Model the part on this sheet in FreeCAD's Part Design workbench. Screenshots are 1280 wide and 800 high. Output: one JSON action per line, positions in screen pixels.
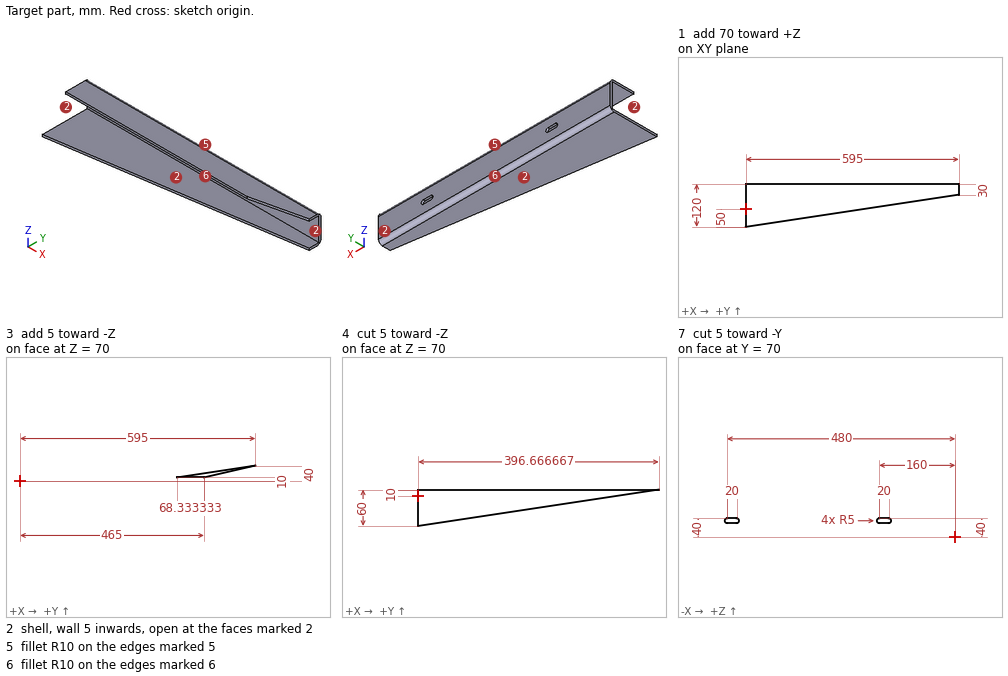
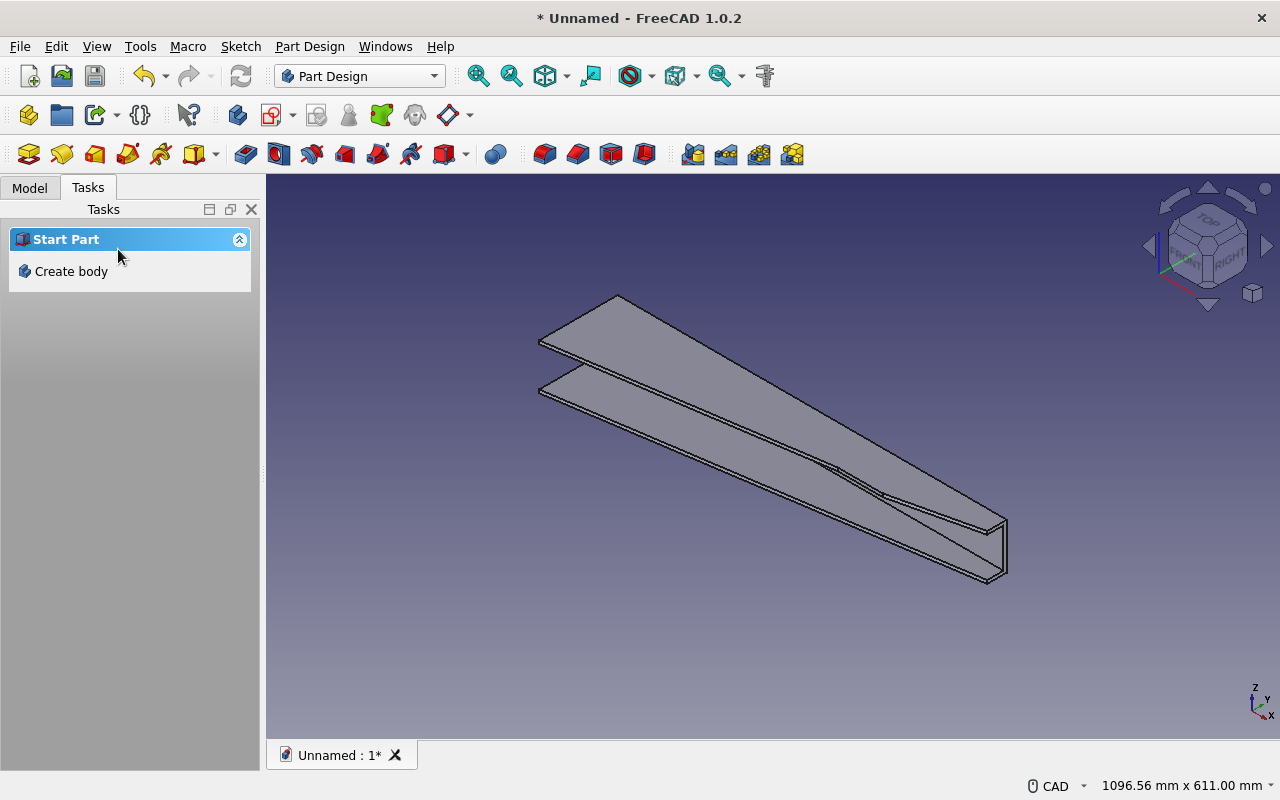
{"action": "left_click", "coordinate": [729, 391]}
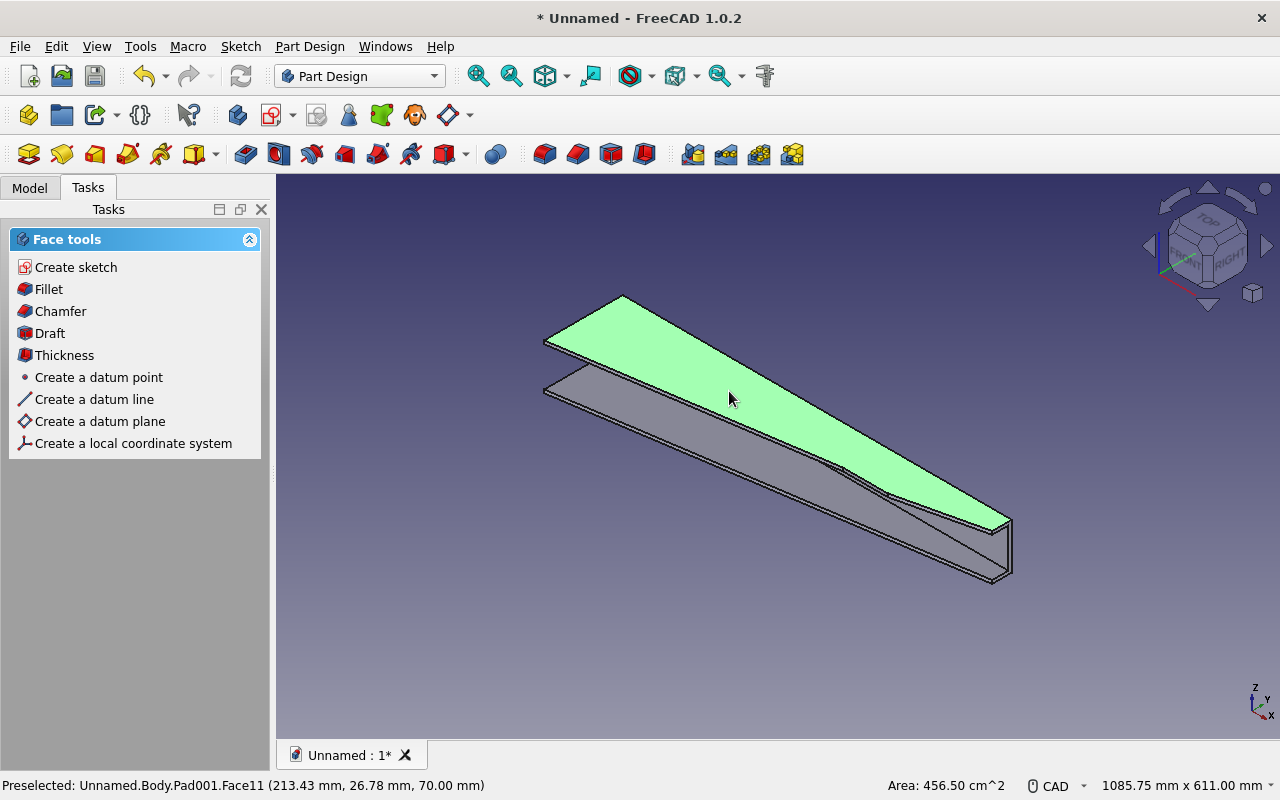
{"action": "left_click", "coordinate": [270, 116]}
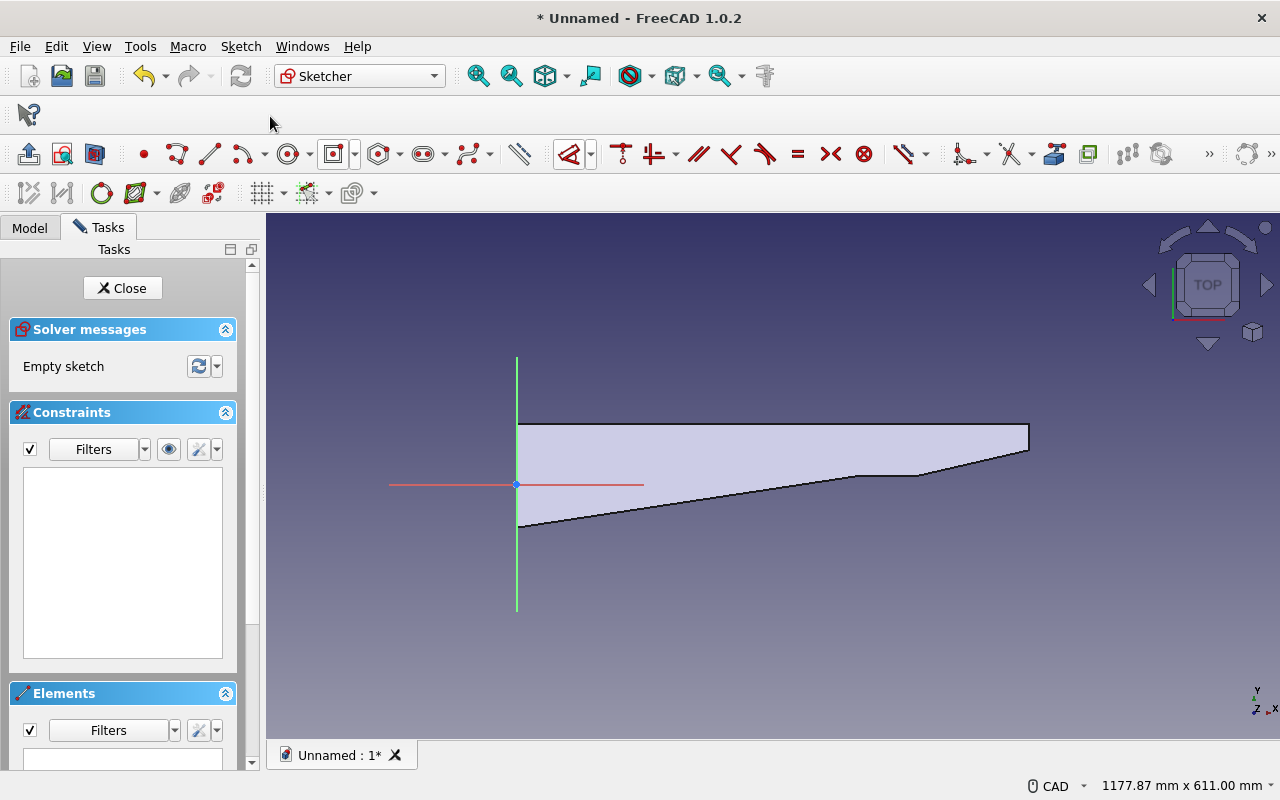
{"action": "scroll", "coordinate": [667, 533], "scroll_direction": "up", "scroll_amount": 3}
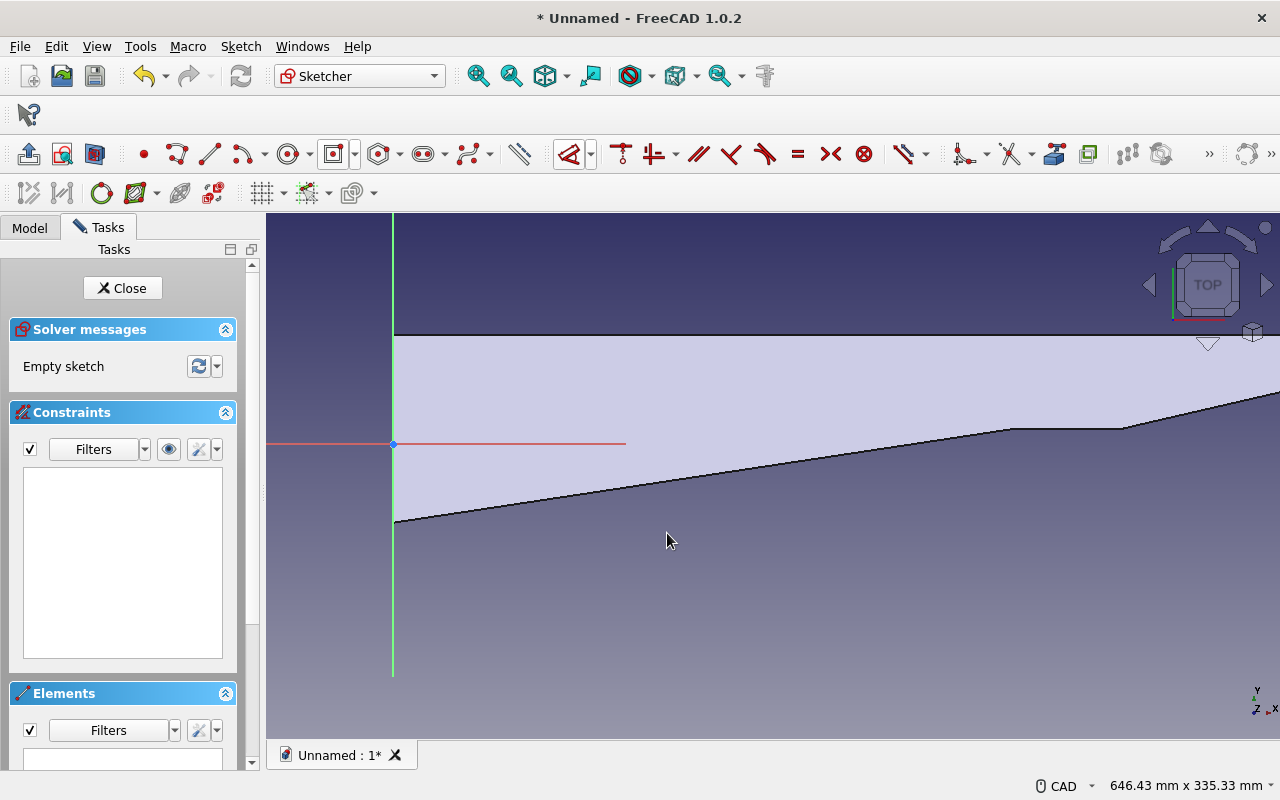
{"action": "left_click", "coordinate": [177, 154]}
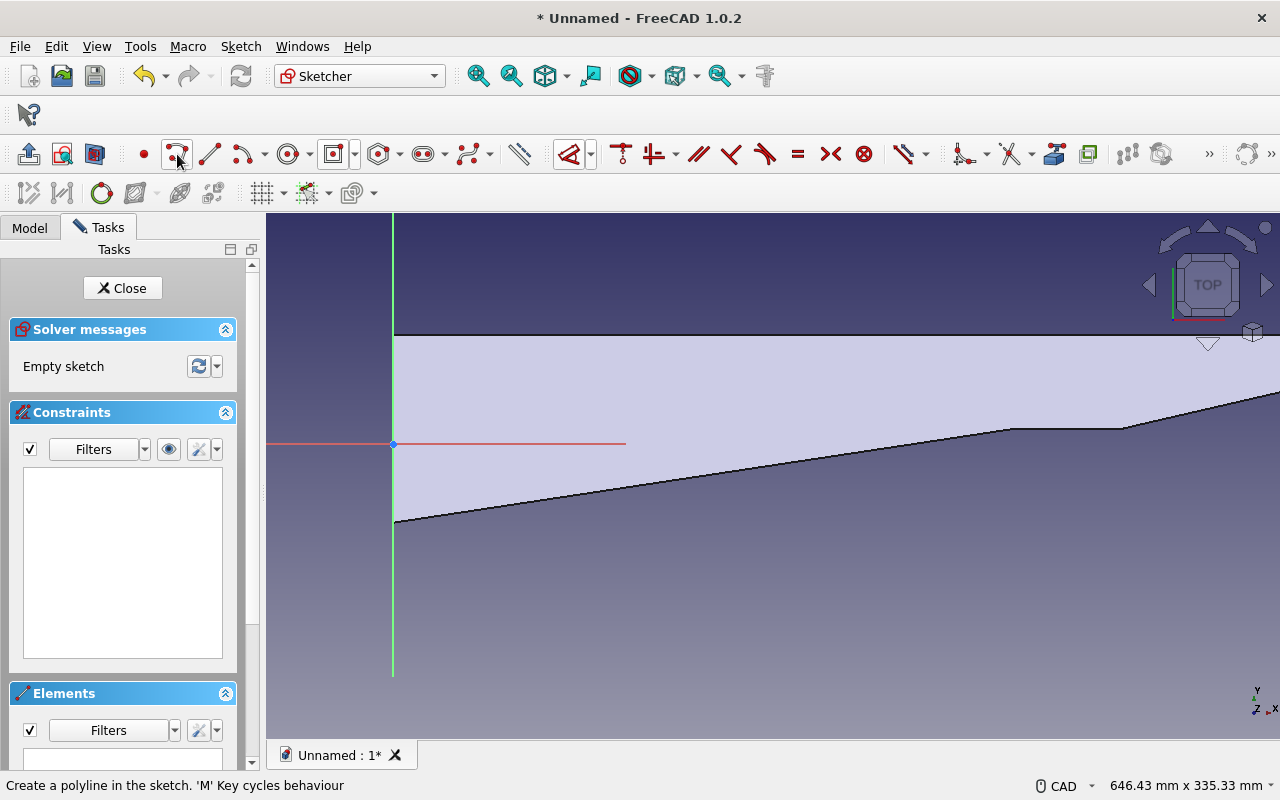
{"action": "left_click", "coordinate": [393, 429]}
{"action": "left_click", "coordinate": [402, 523]}
{"action": "left_click", "coordinate": [1015, 429]}
{"action": "left_click", "coordinate": [393, 430]}
{"action": "key", "text": "Escape"}
{"action": "key", "text": "Escape"}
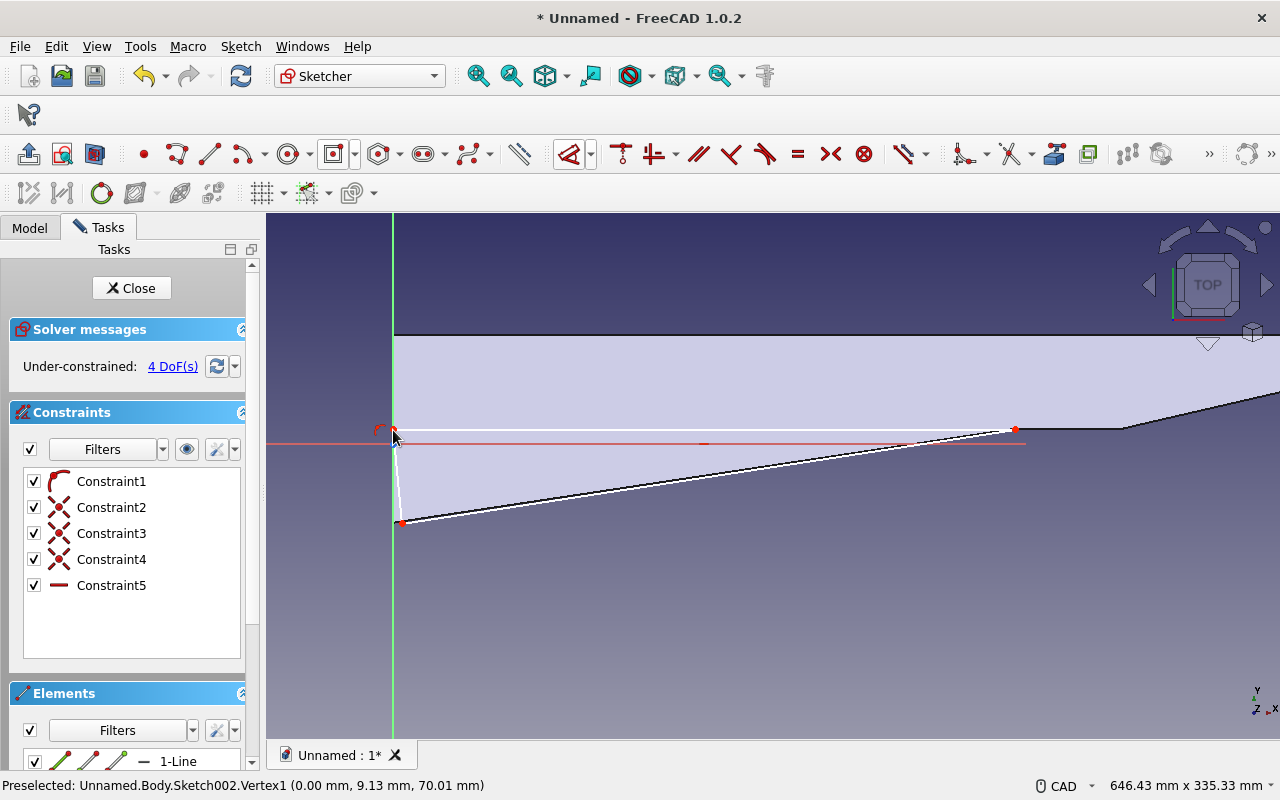
{"action": "left_click", "coordinate": [396, 458]}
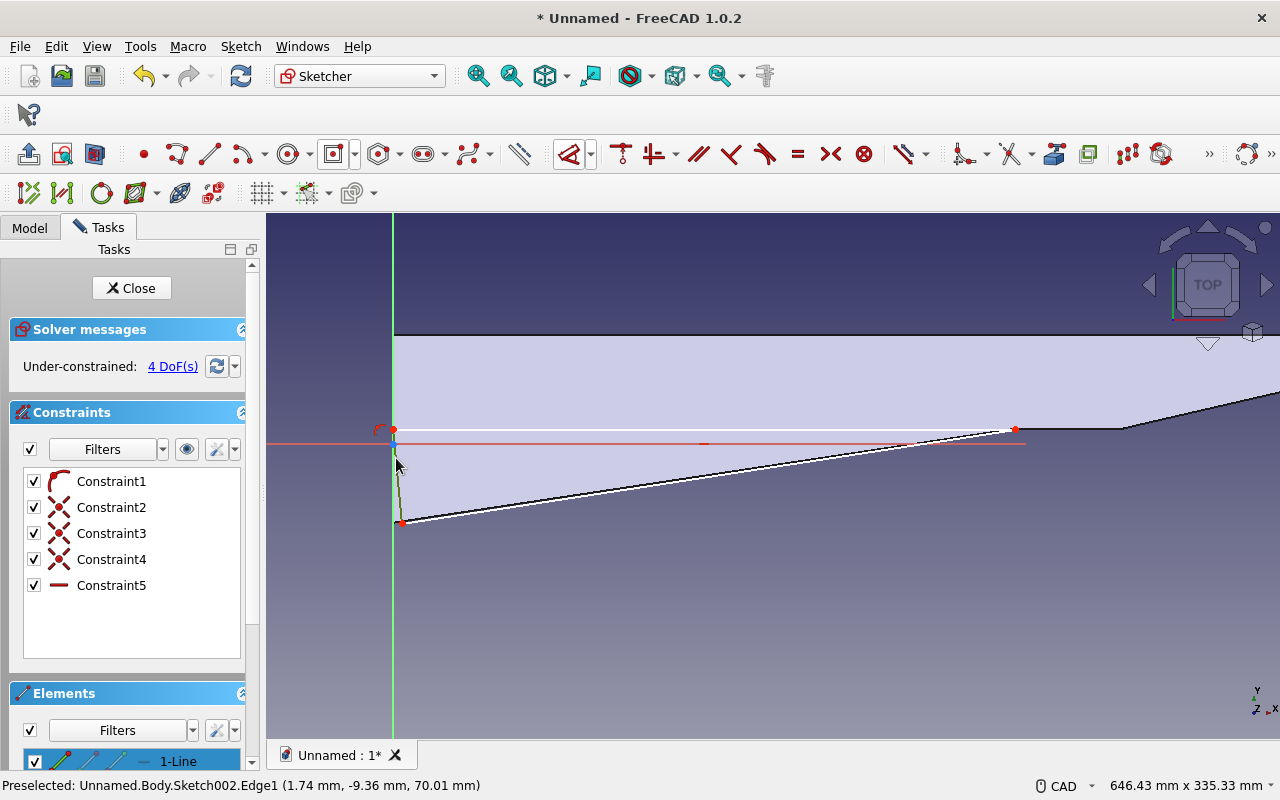
{"action": "key", "text": "v"}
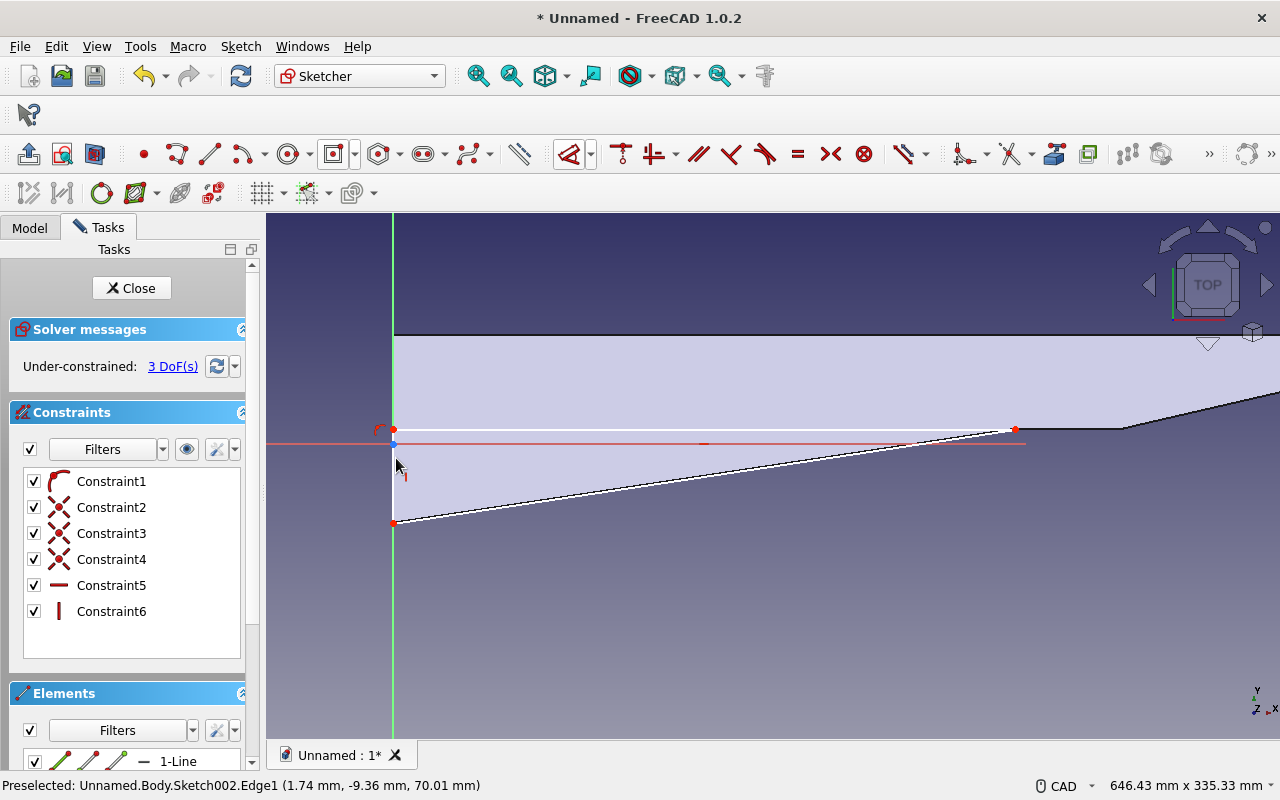
{"action": "left_click", "coordinate": [393, 458]}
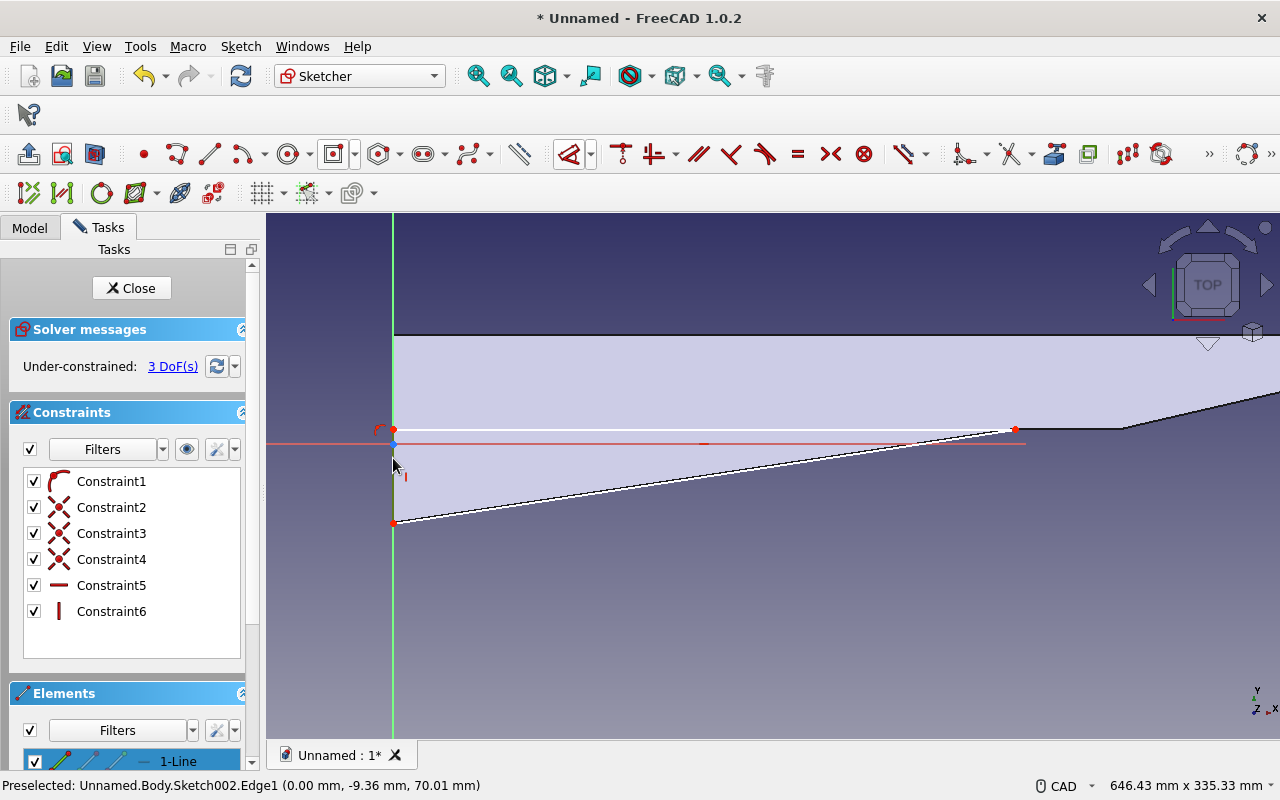
{"action": "key", "text": "i"}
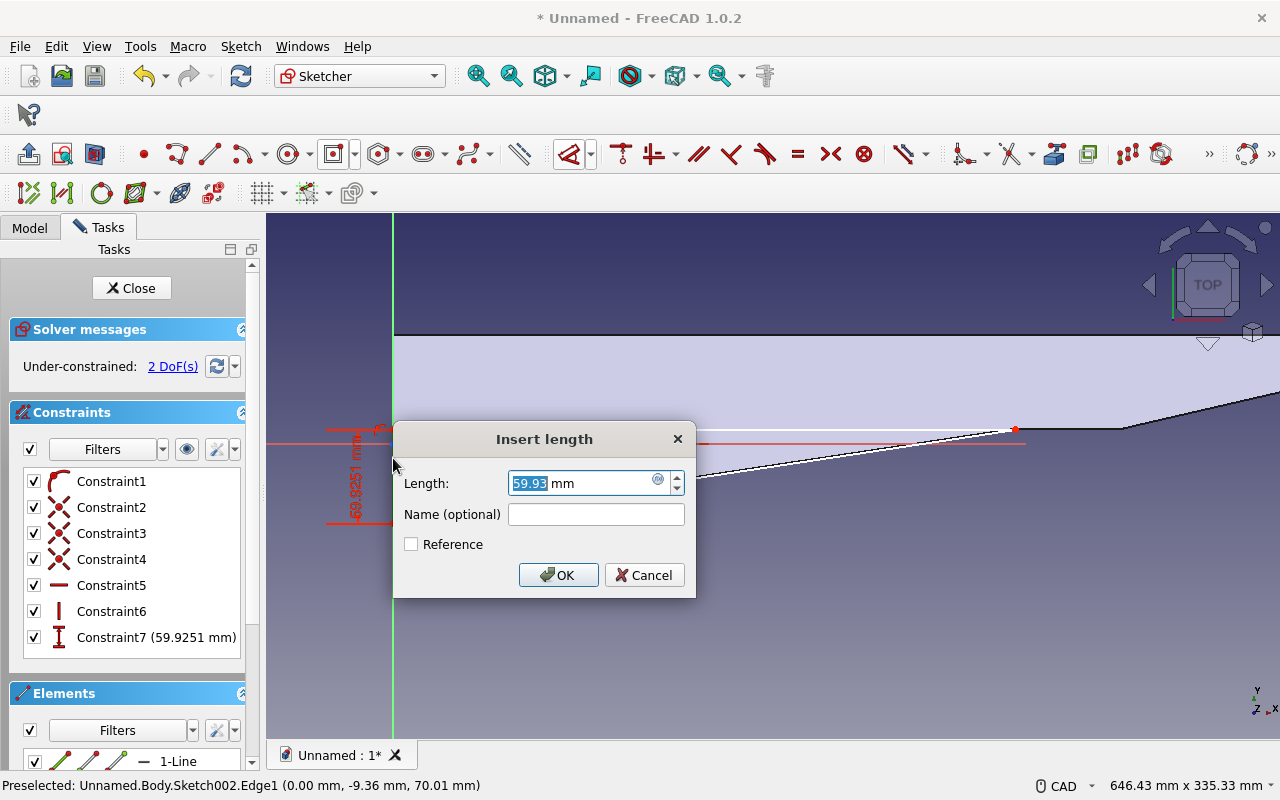
{"action": "type", "text": "60"}
{"action": "key", "text": "Return"}